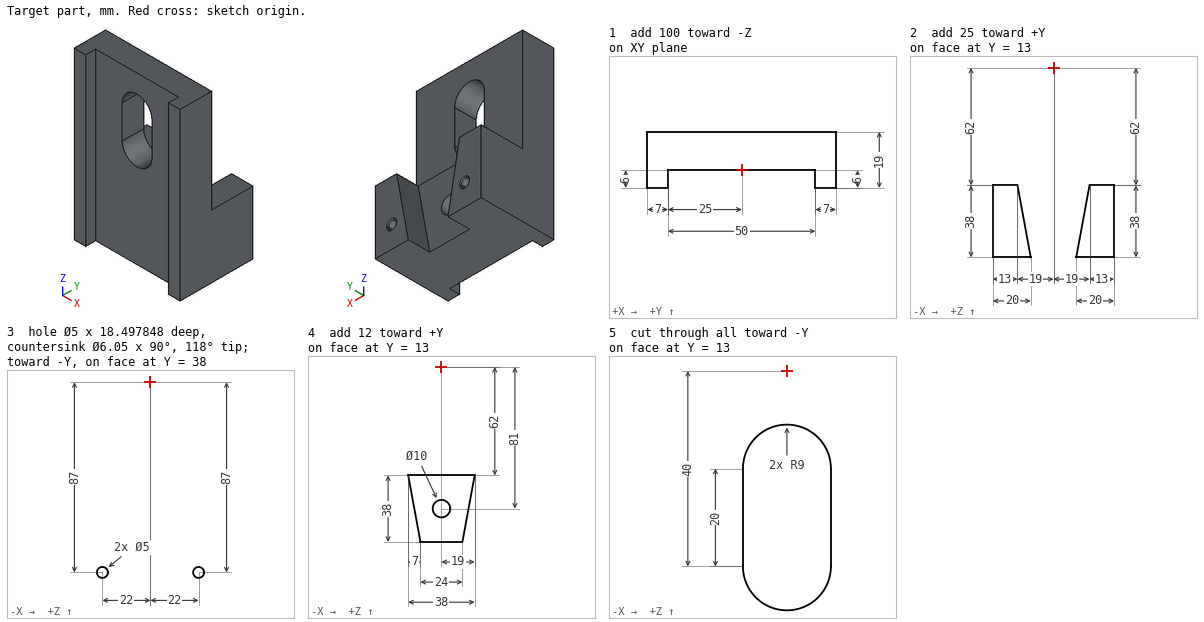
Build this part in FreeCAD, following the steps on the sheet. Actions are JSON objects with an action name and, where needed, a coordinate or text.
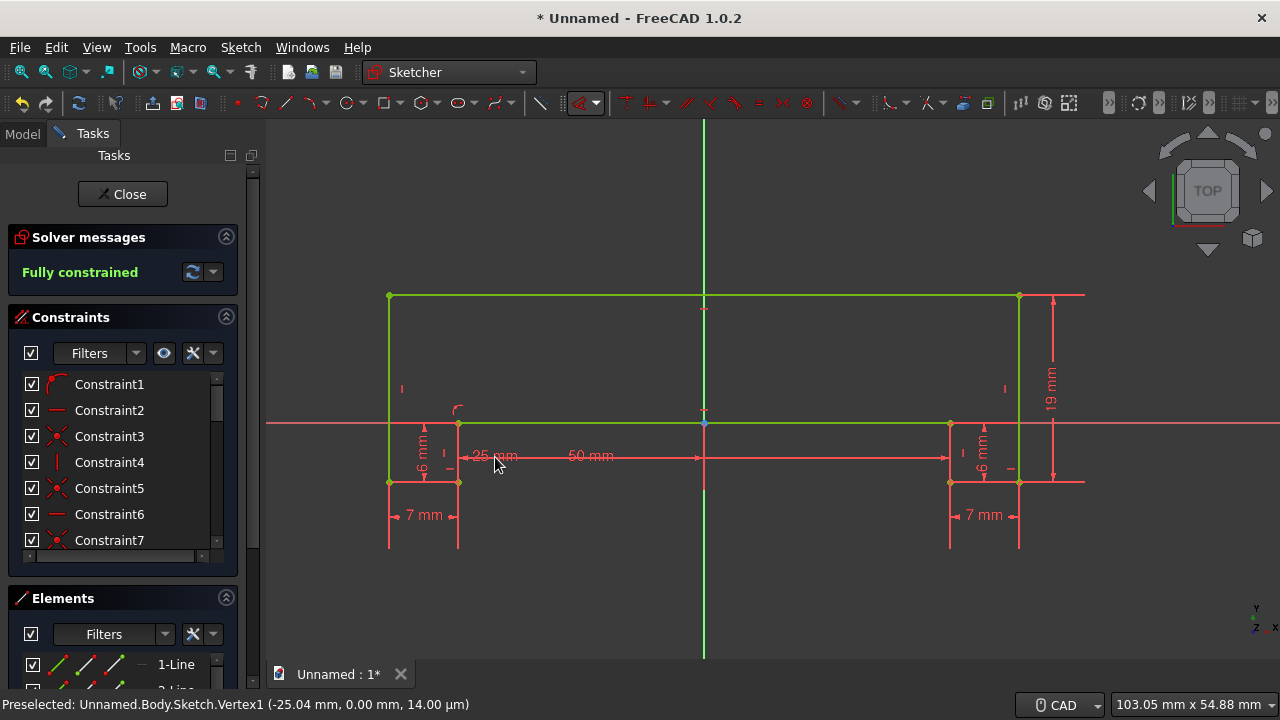
{"action": "left_click", "coordinate": [123, 194]}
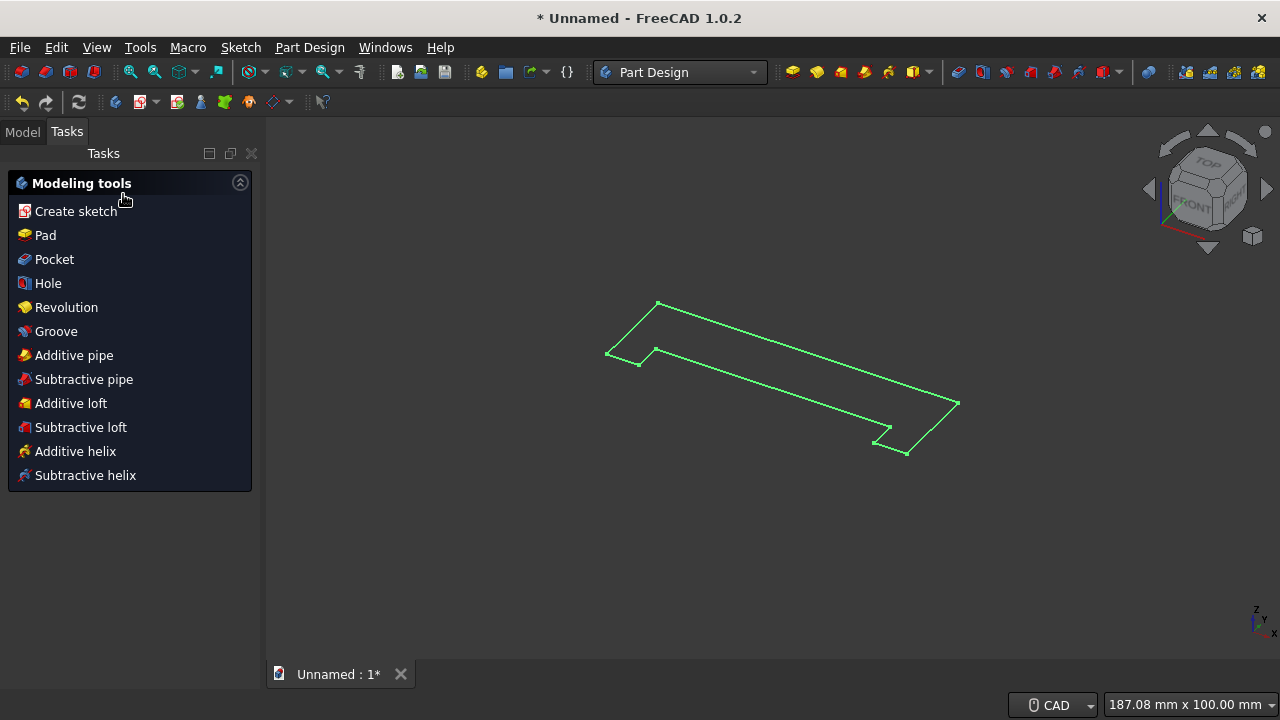
{"action": "left_click", "coordinate": [794, 72]}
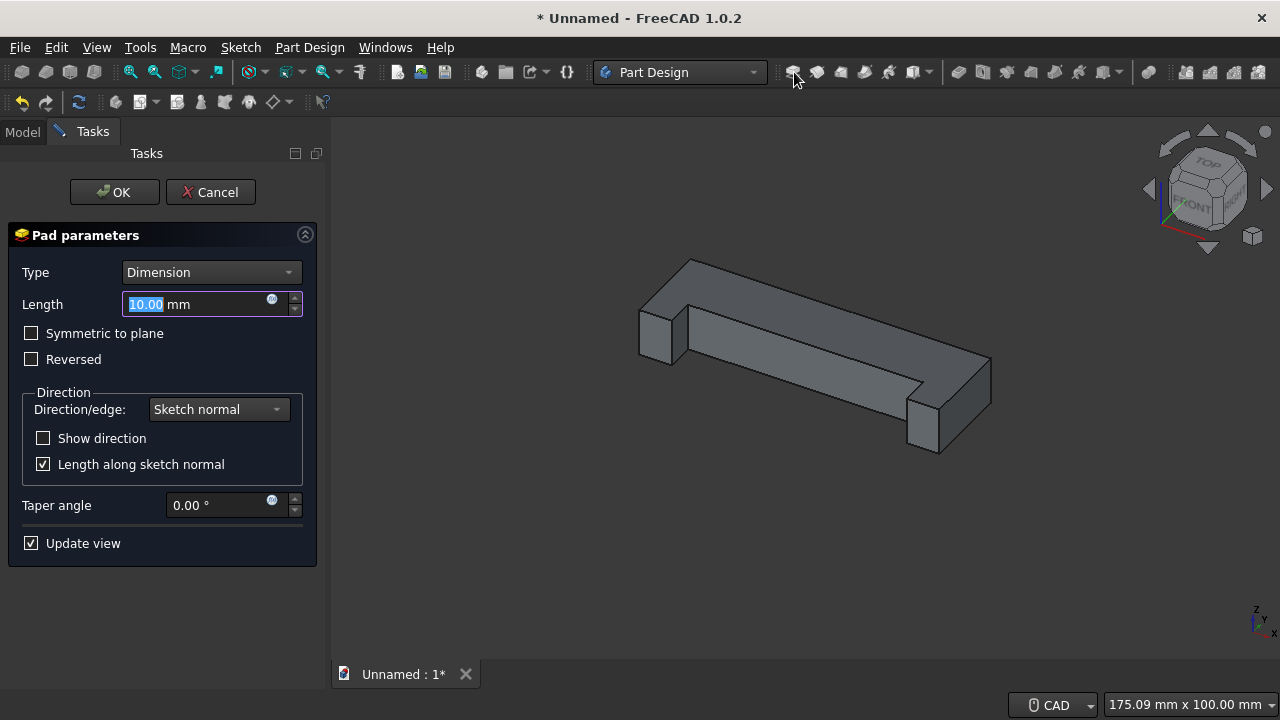
{"action": "type", "text": "100"}
{"action": "key", "text": "Tab"}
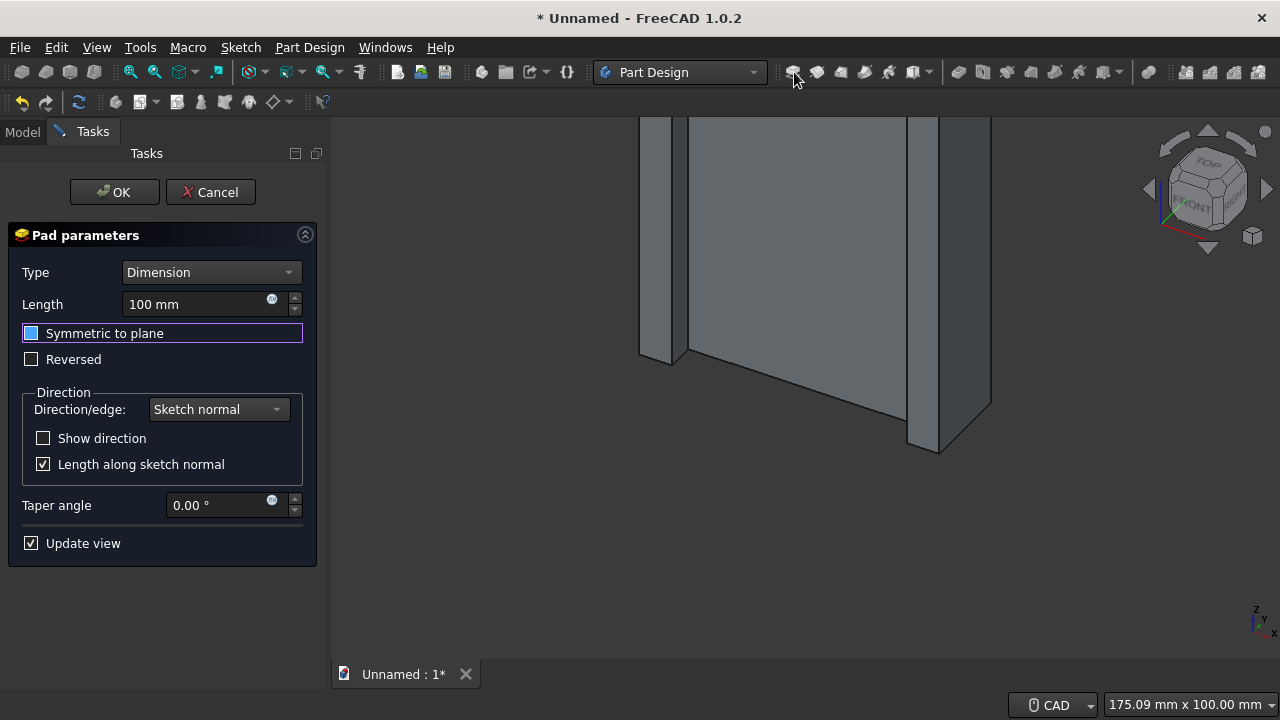
{"action": "left_click", "coordinate": [30, 359]}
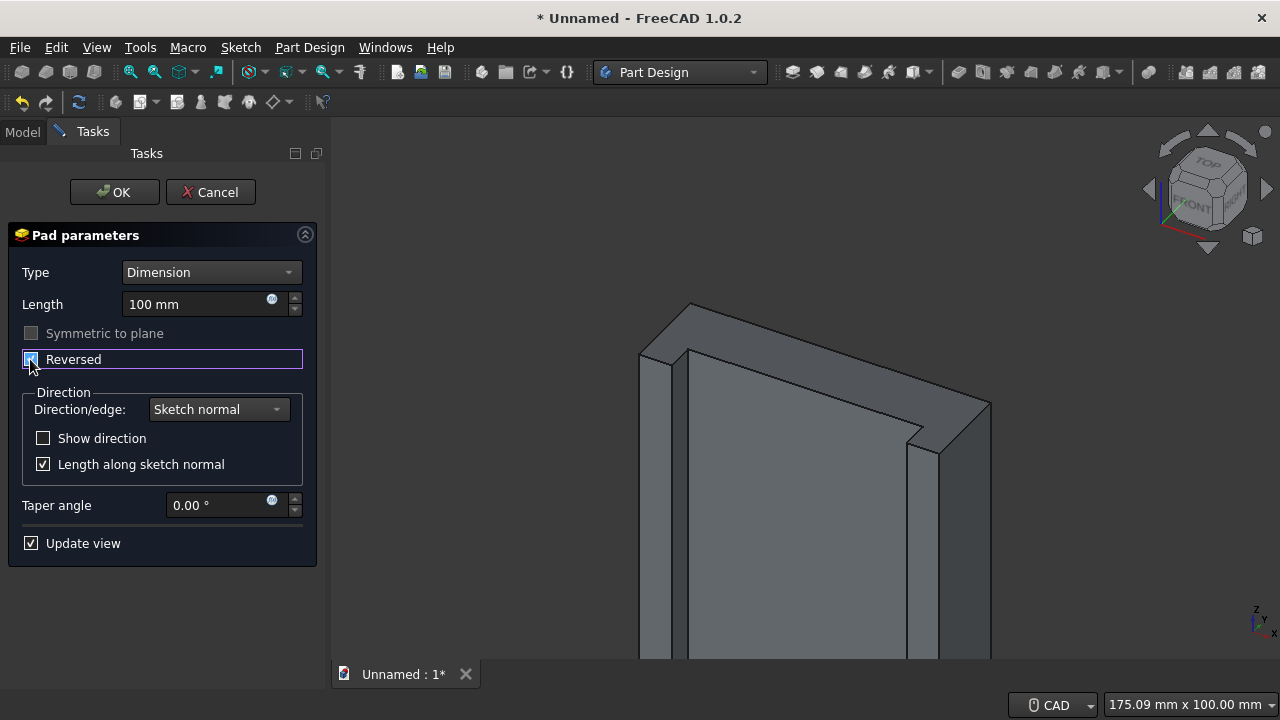
{"action": "left_click", "coordinate": [115, 192]}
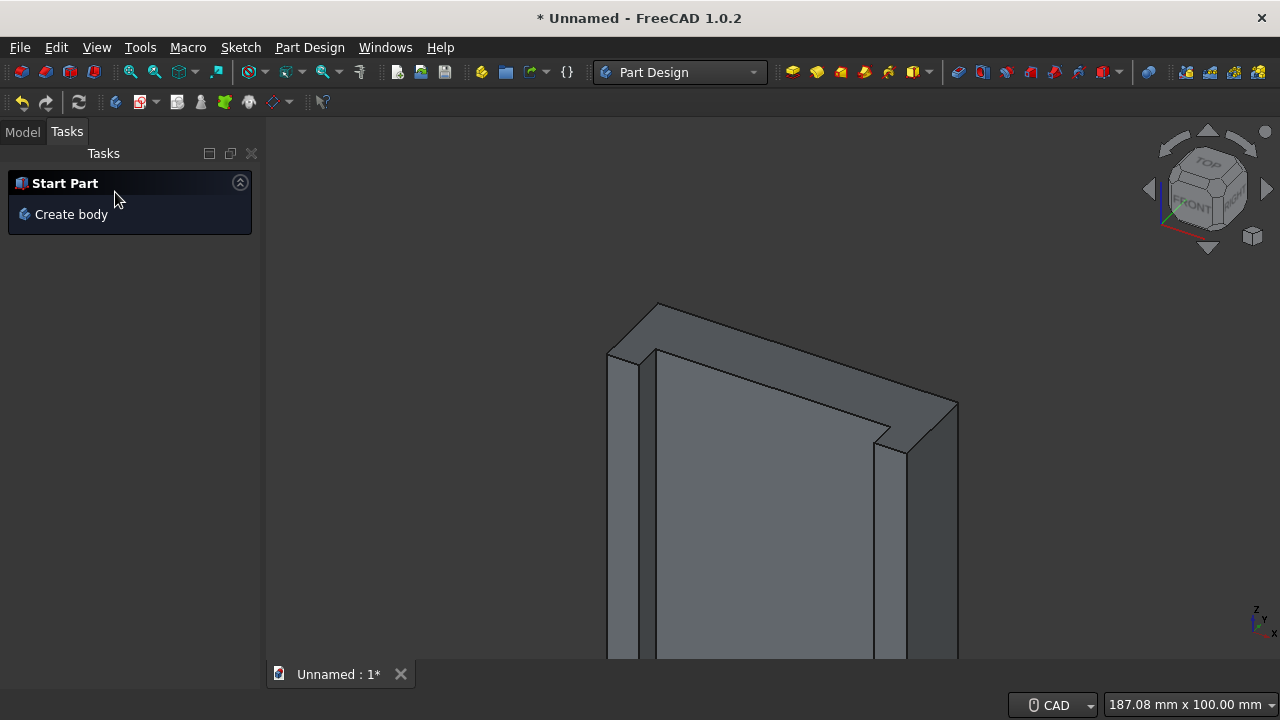
{"action": "key", "text": "v f"}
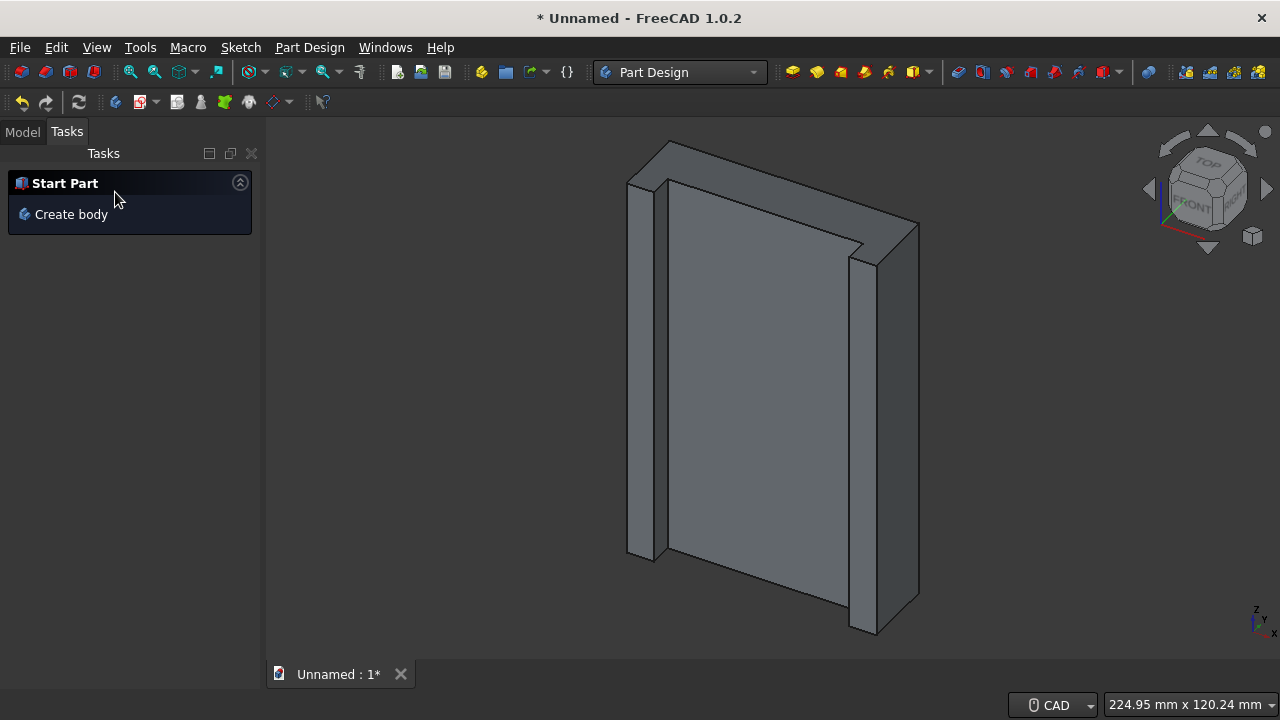
{"action": "key", "text": "4"}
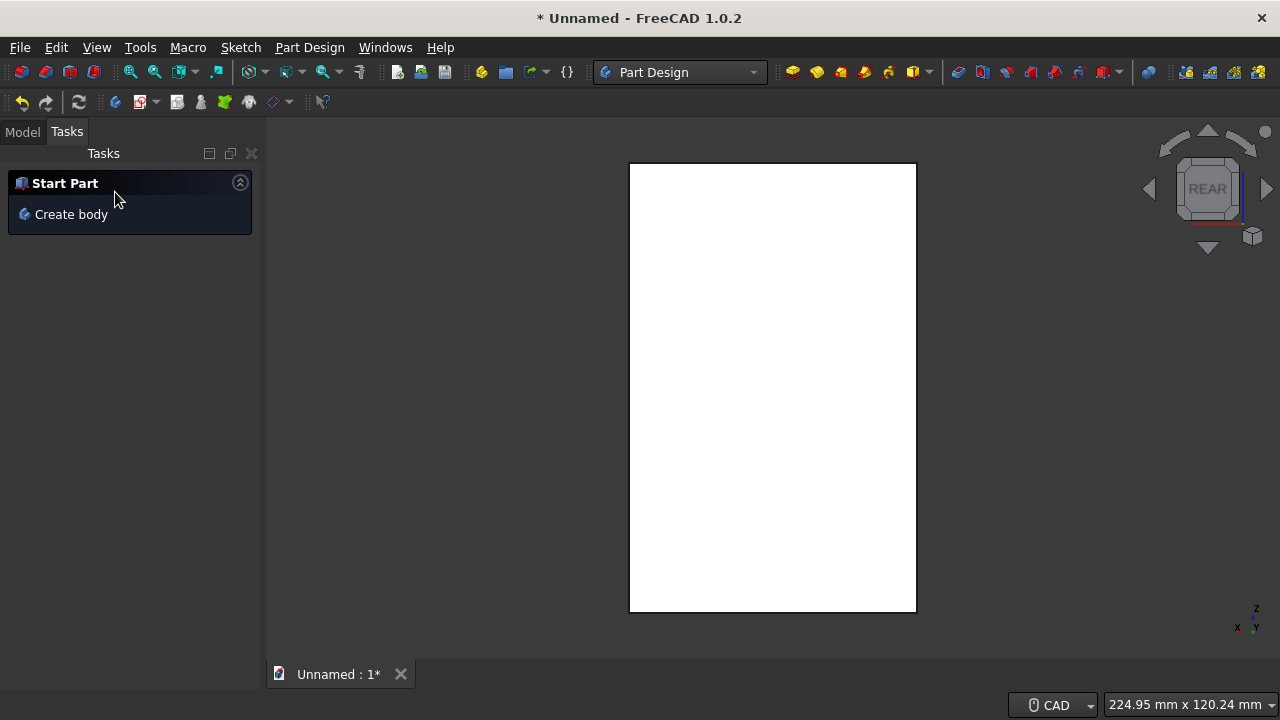
{"action": "left_click", "coordinate": [773, 323]}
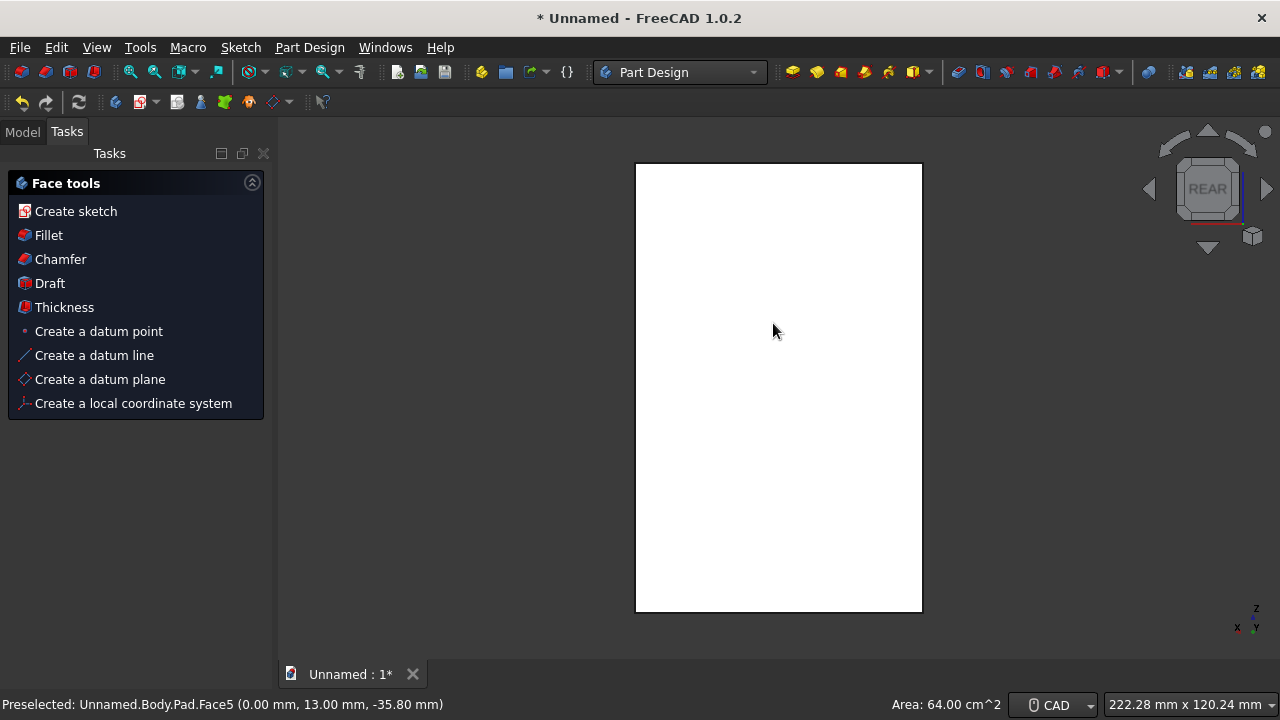
{"action": "left_click", "coordinate": [140, 102]}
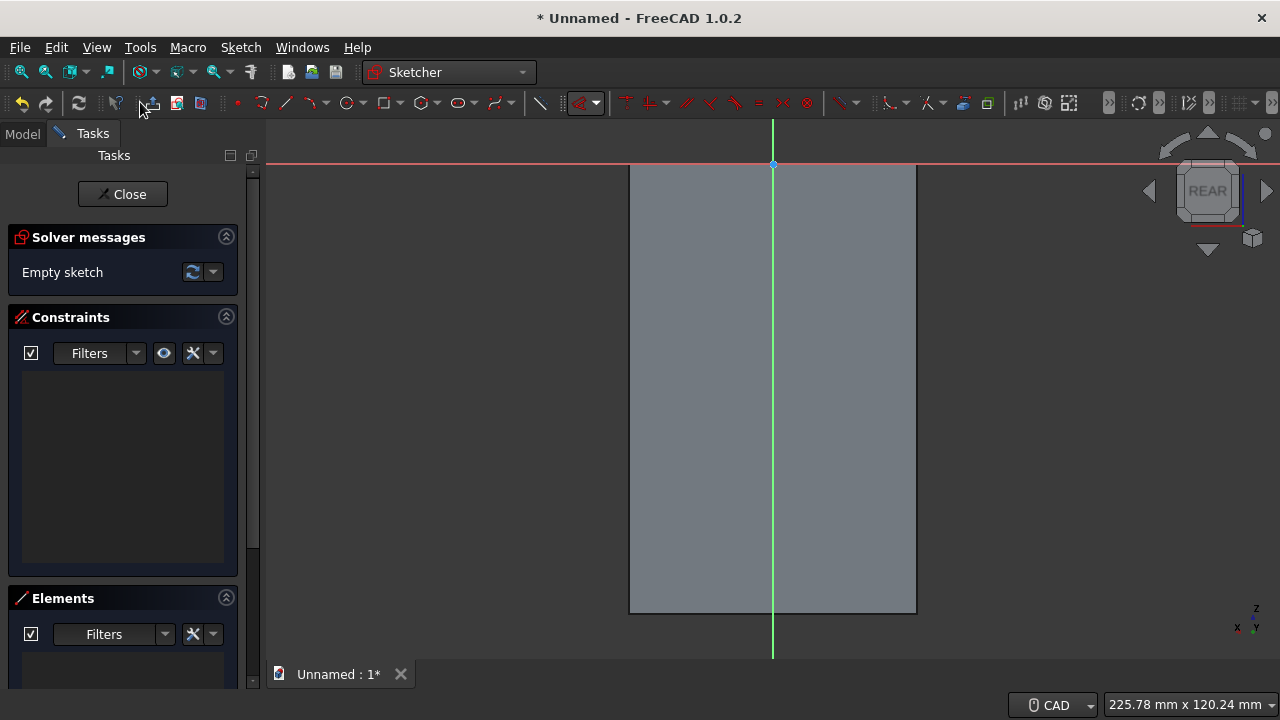
{"action": "scroll", "coordinate": [395, 389], "scroll_direction": "down", "scroll_amount": 1}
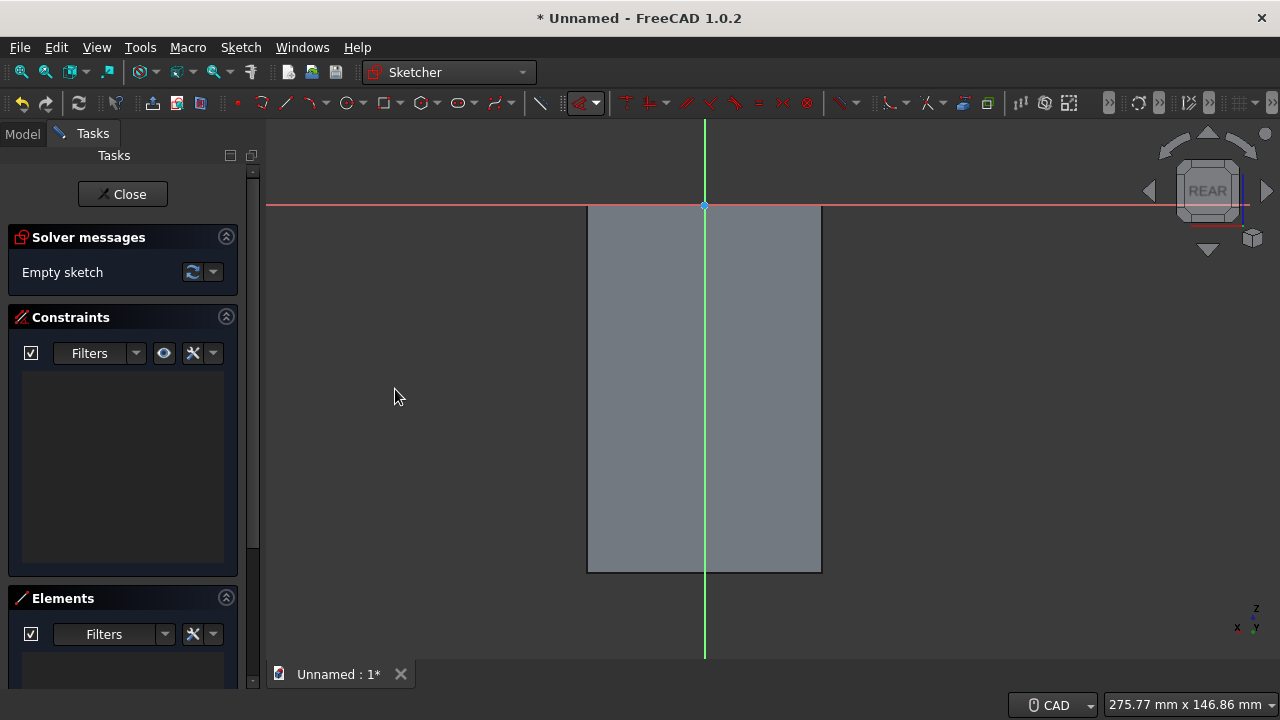
{"action": "key", "text": "g m"}